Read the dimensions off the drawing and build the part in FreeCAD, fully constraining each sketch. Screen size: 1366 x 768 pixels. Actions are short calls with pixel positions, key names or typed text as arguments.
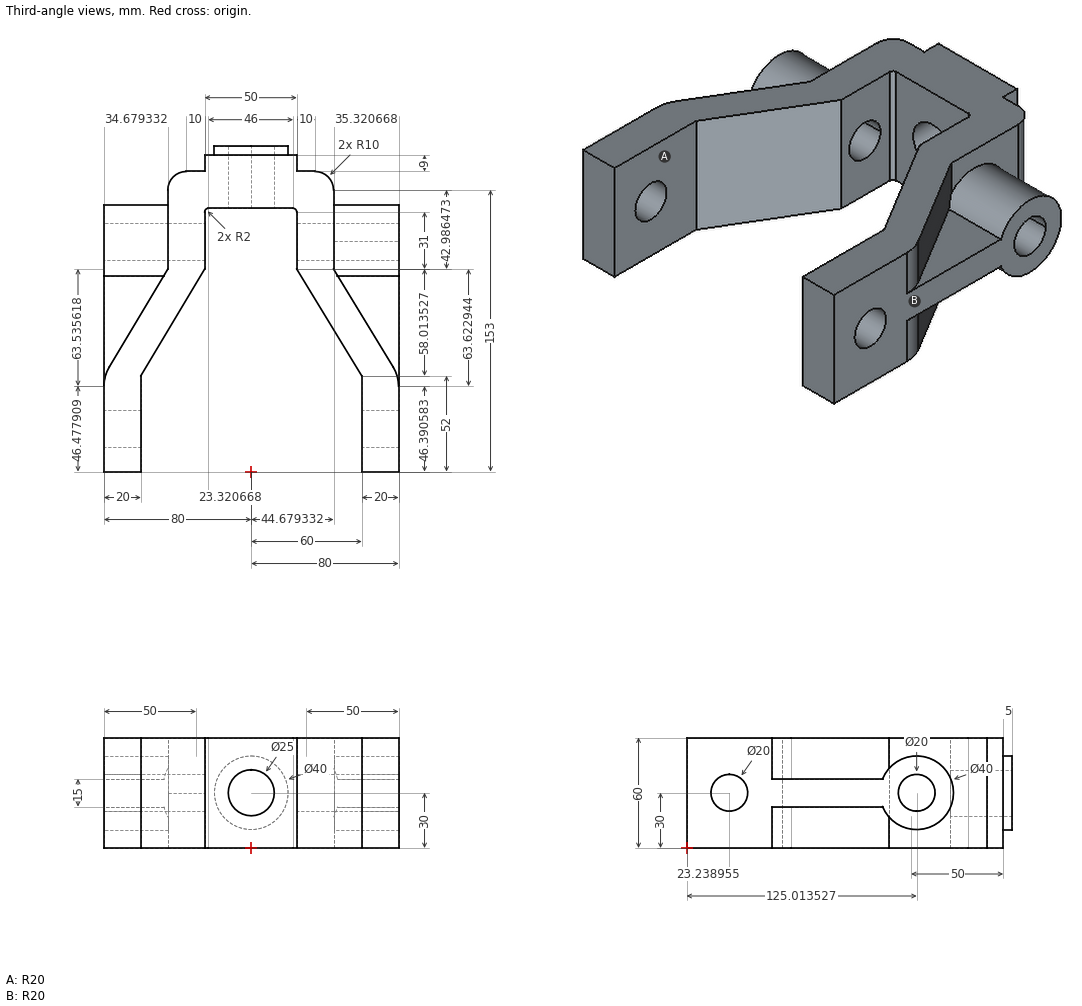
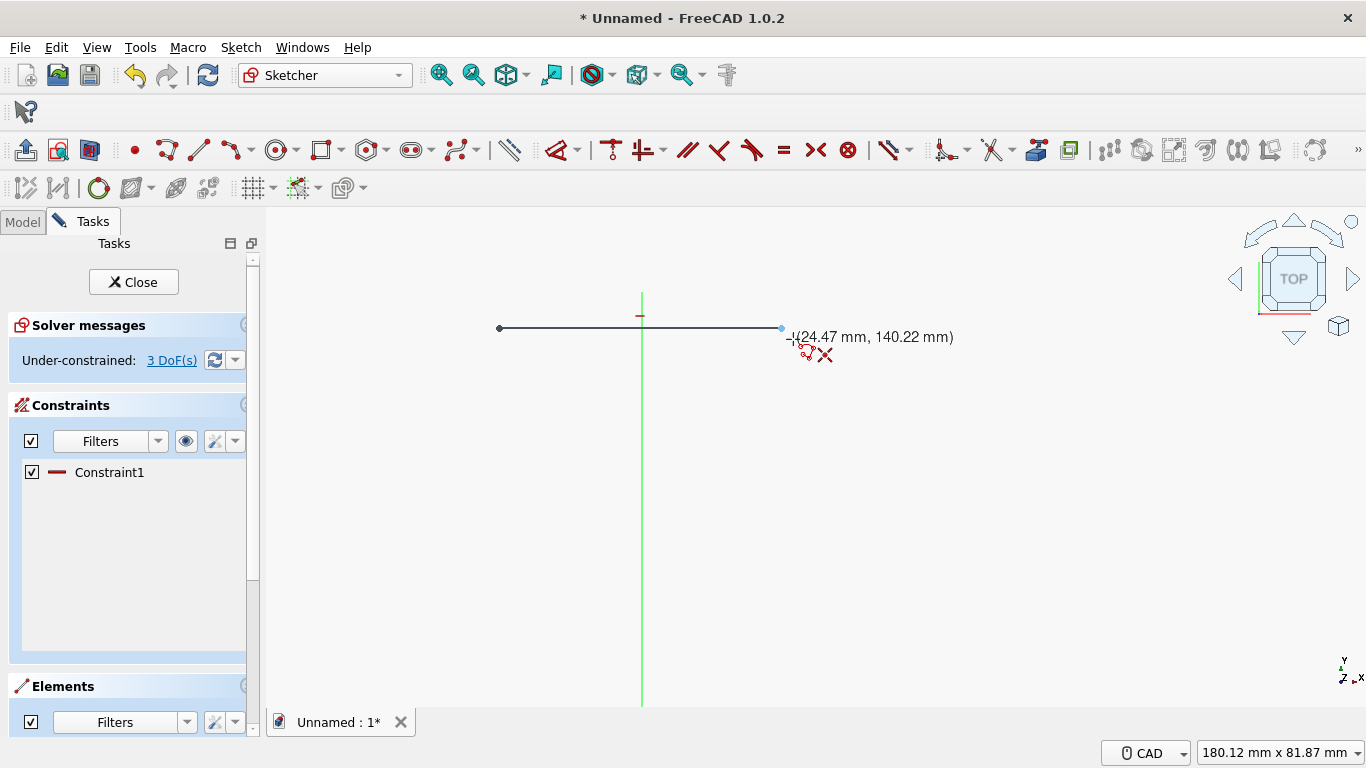
click(793, 337)
click(793, 526)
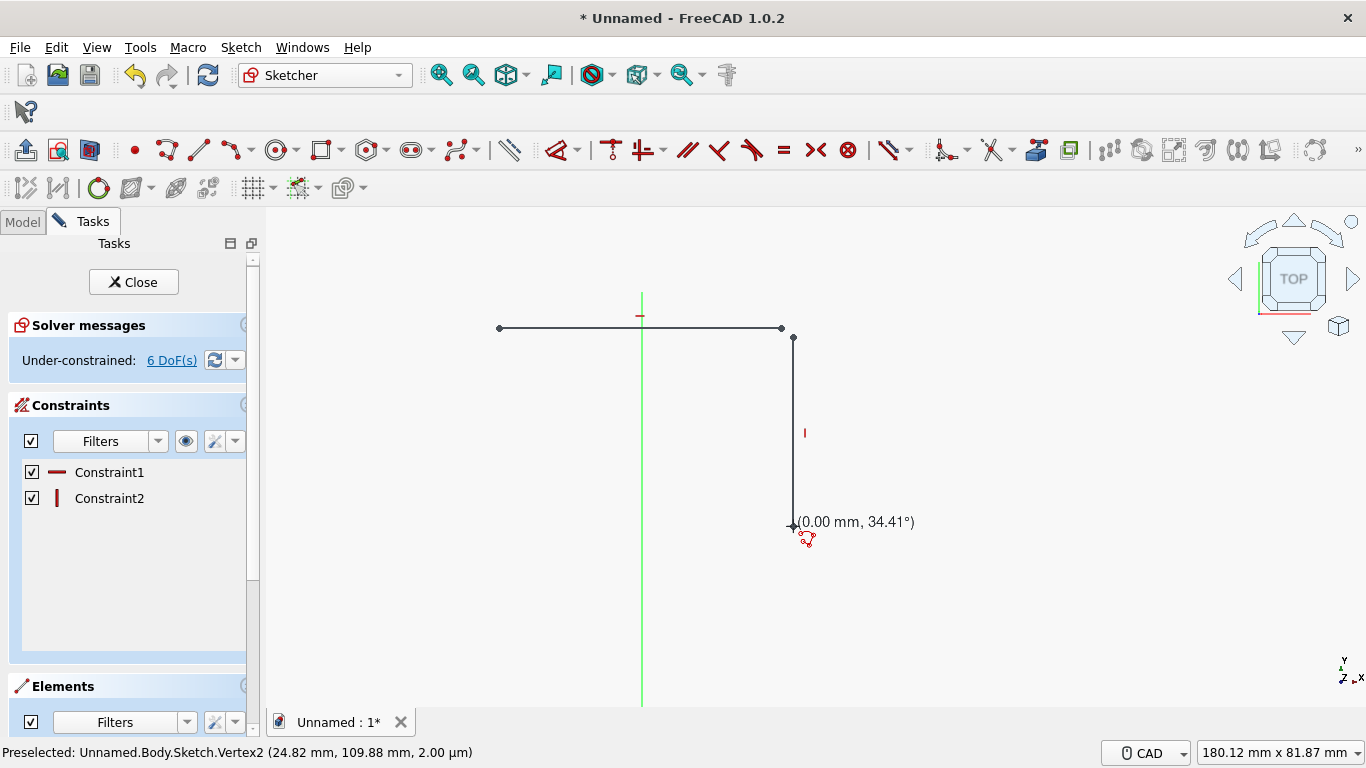
scroll(793, 364, down, 6)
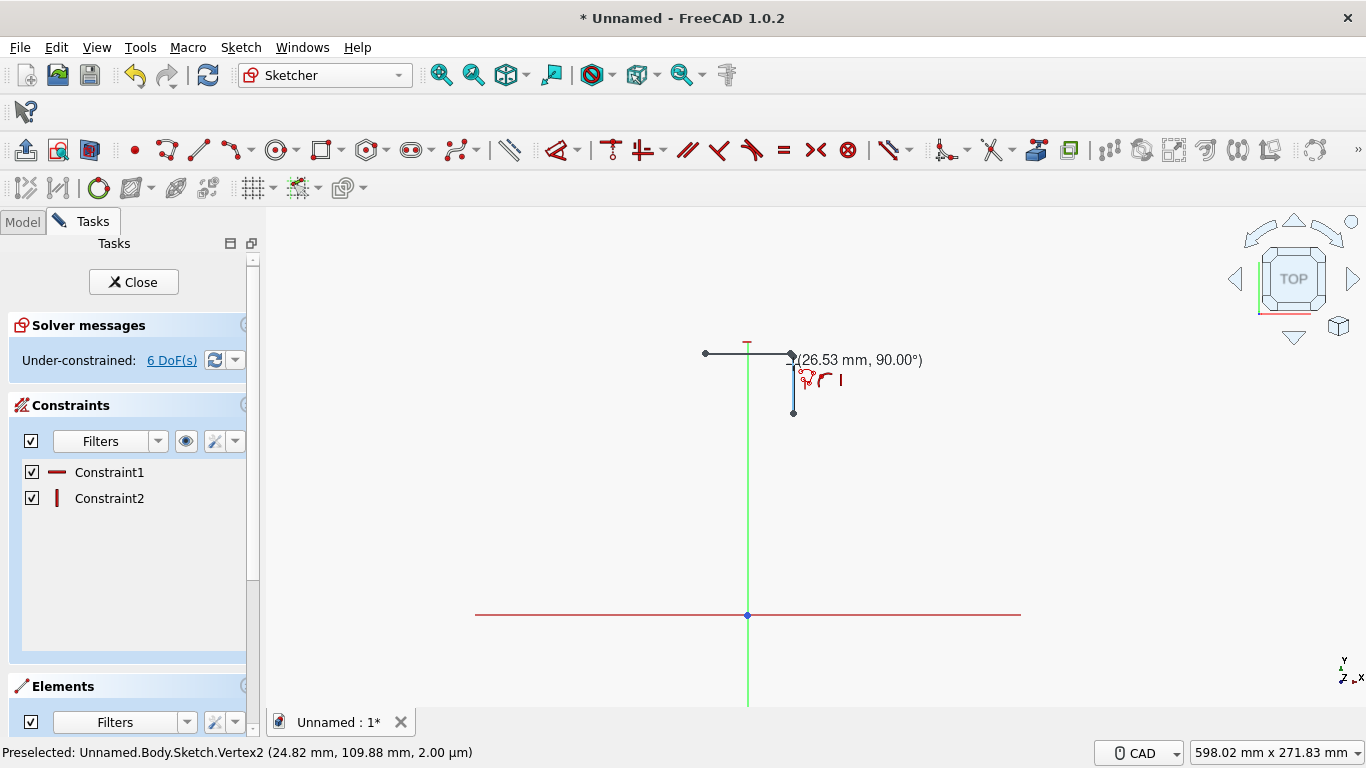
click(858, 520)
click(858, 615)
click(895, 606)
click(895, 520)
click(830, 413)
click(830, 334)
right_click(830, 334)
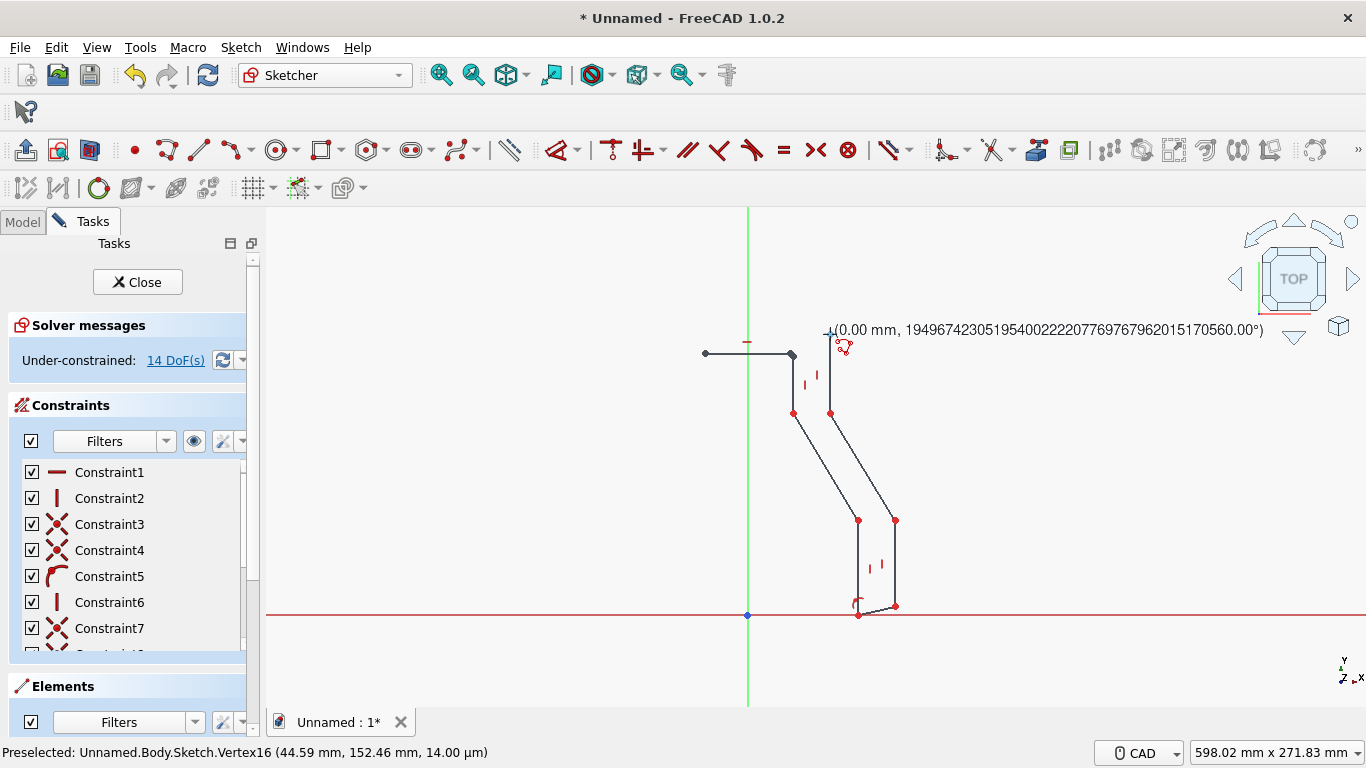
click(812, 316)
click(793, 316)
click(793, 299)
click(701, 299)
click(701, 316)
click(683, 316)
right_click(683, 316)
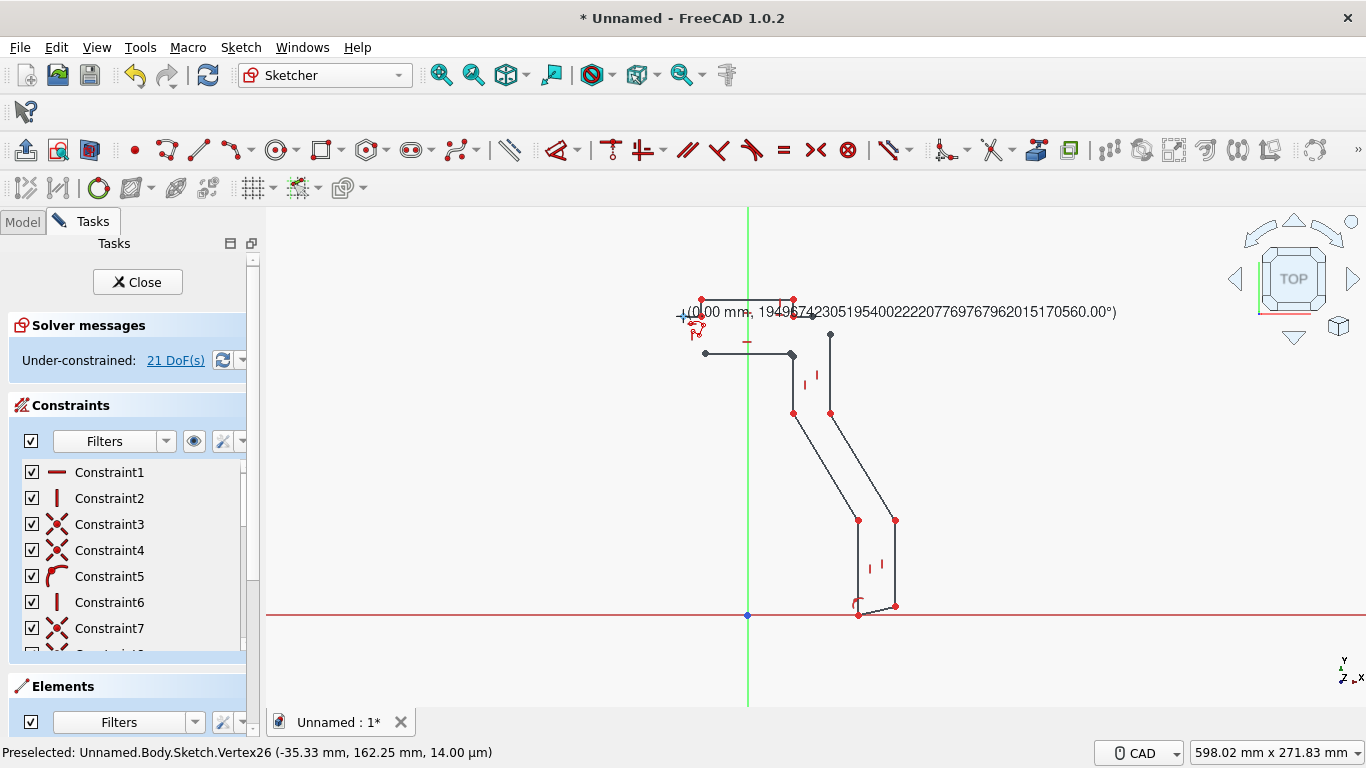
click(665, 334)
click(665, 413)
click(601, 520)
click(601, 615)
click(638, 606)
click(638, 520)
click(701, 413)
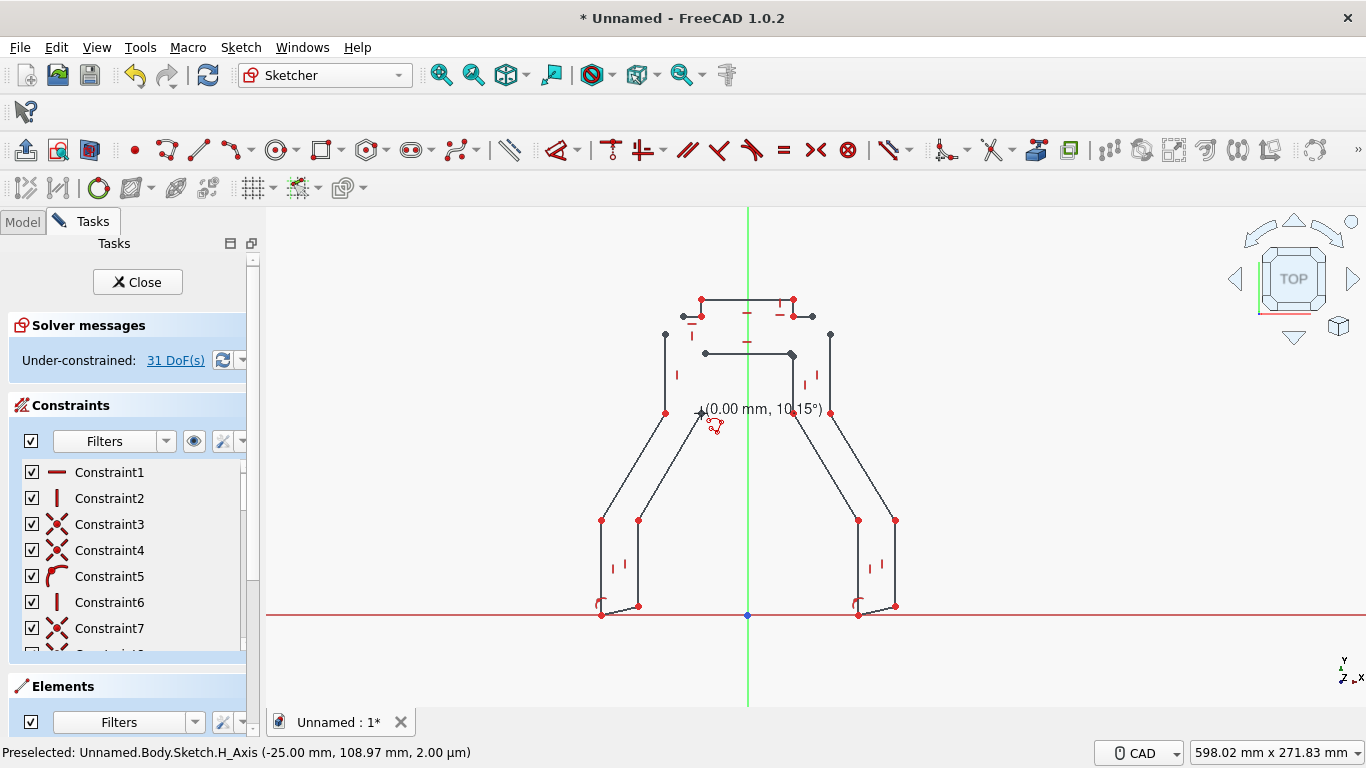
scroll(701, 356, up, 6)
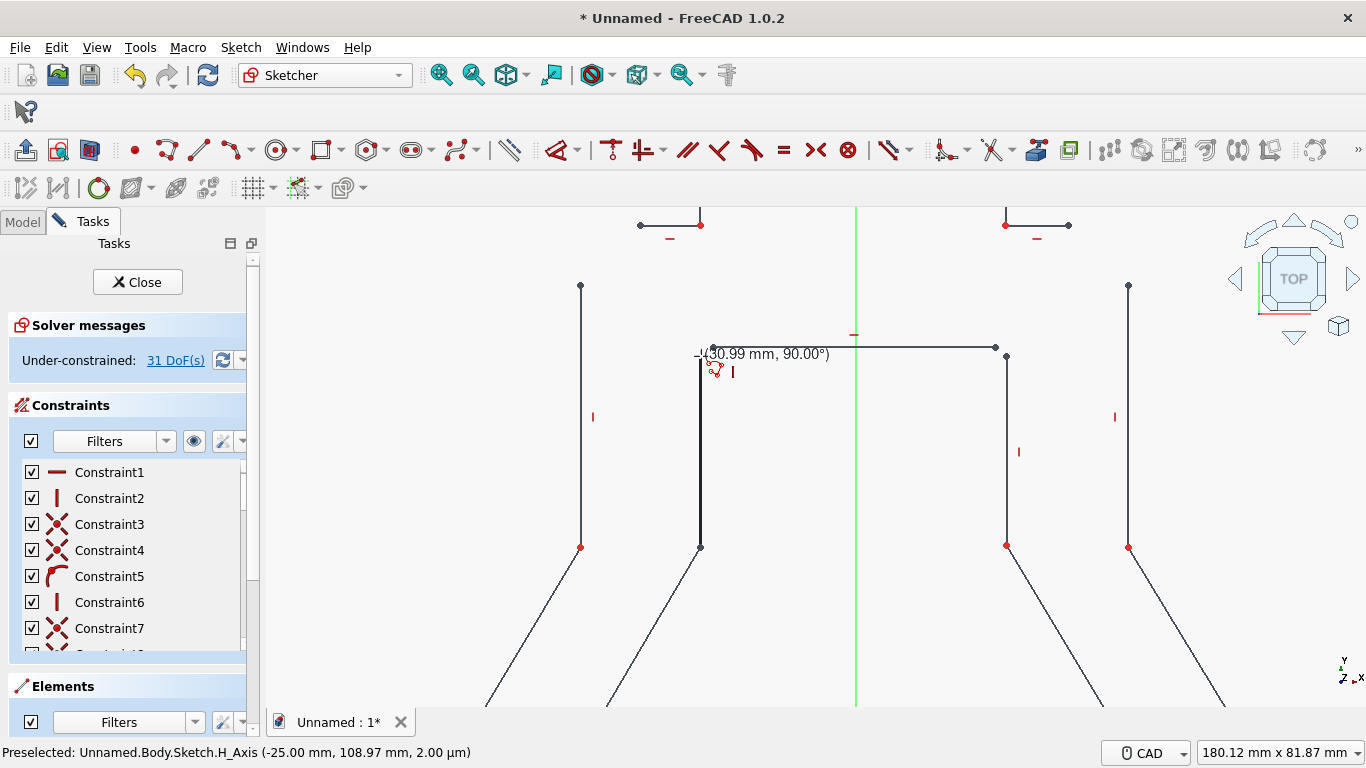
click(700, 355)
right_click(700, 355)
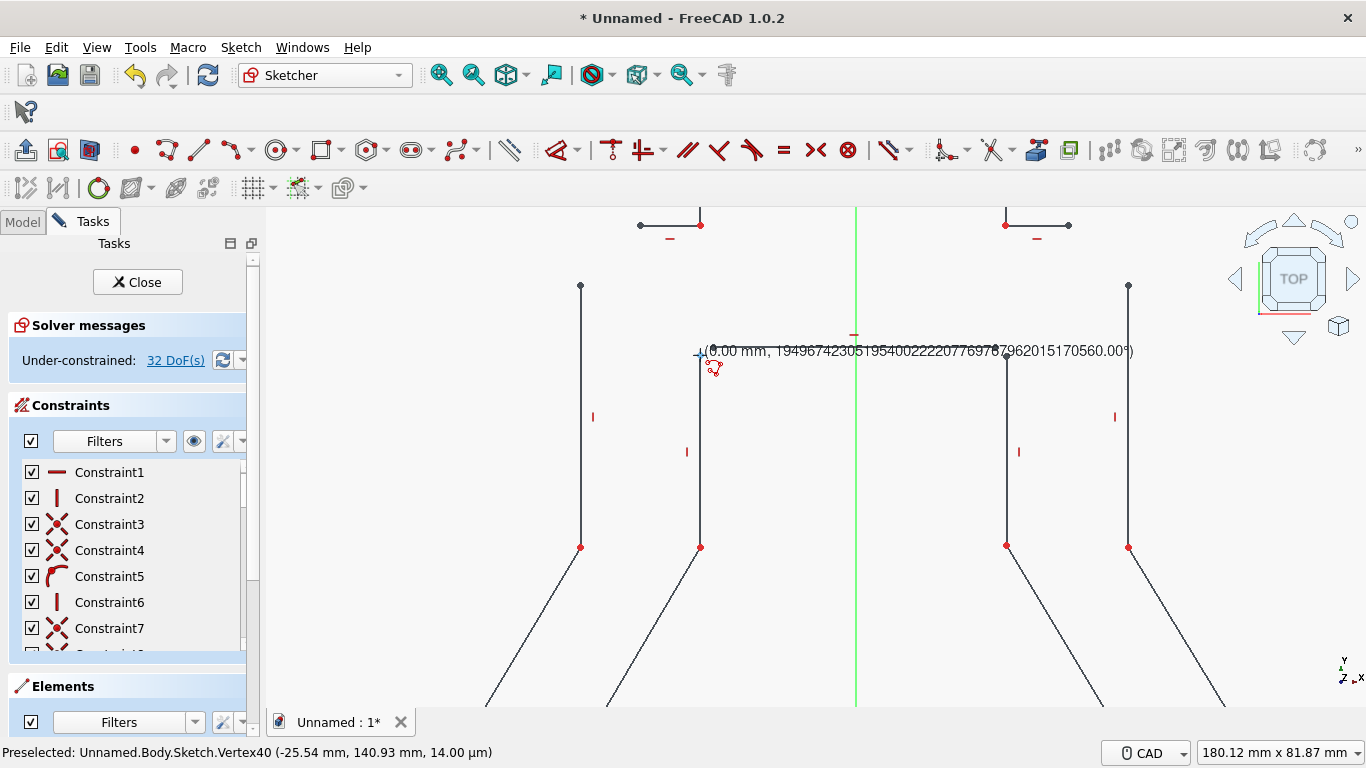
click(232, 150)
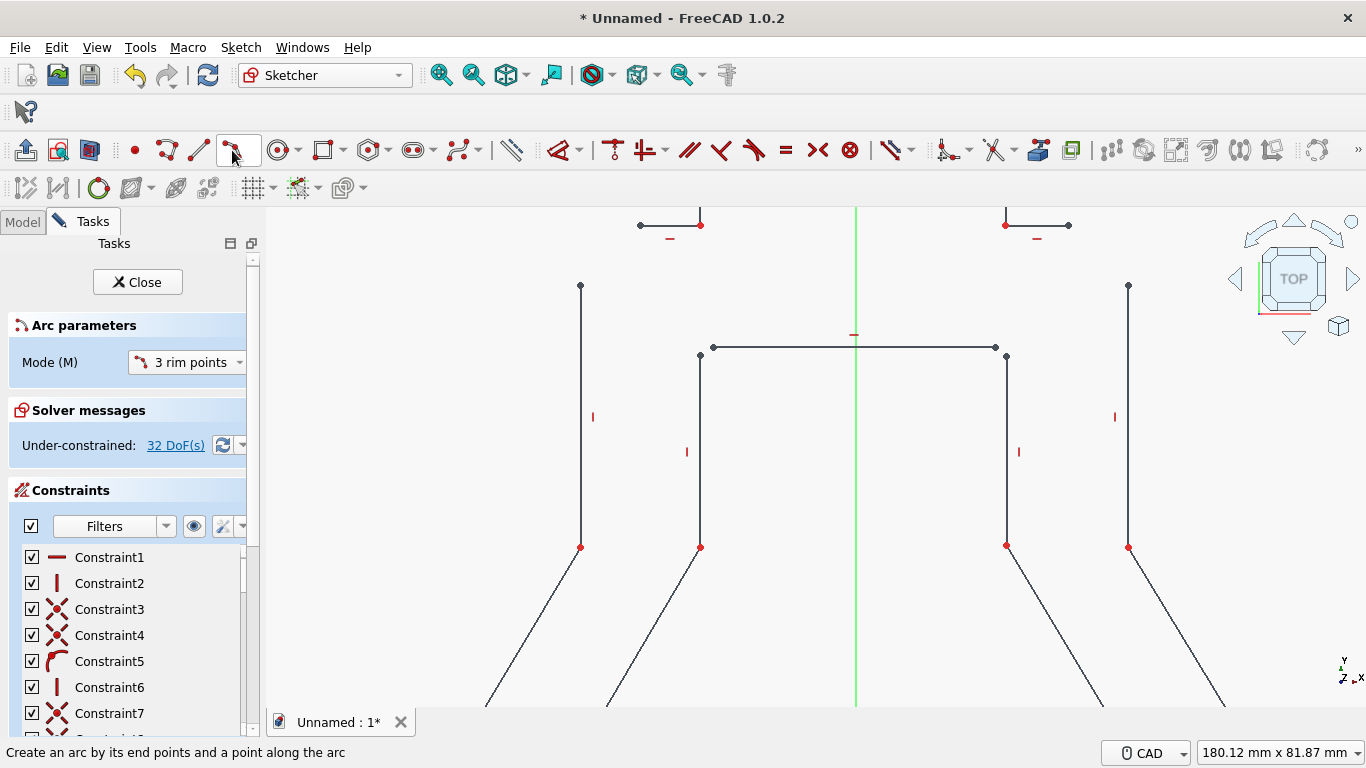
click(996, 347)
click(1007, 357)